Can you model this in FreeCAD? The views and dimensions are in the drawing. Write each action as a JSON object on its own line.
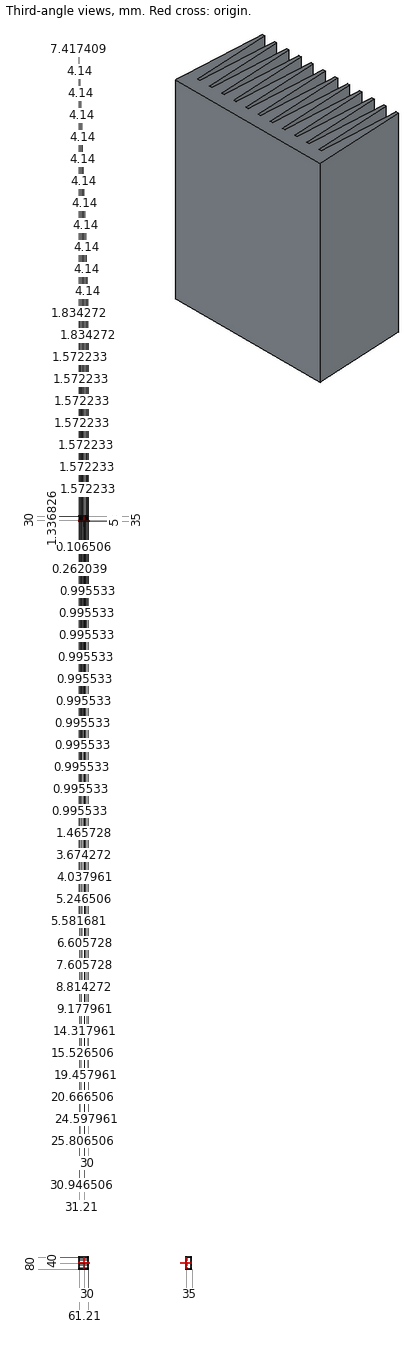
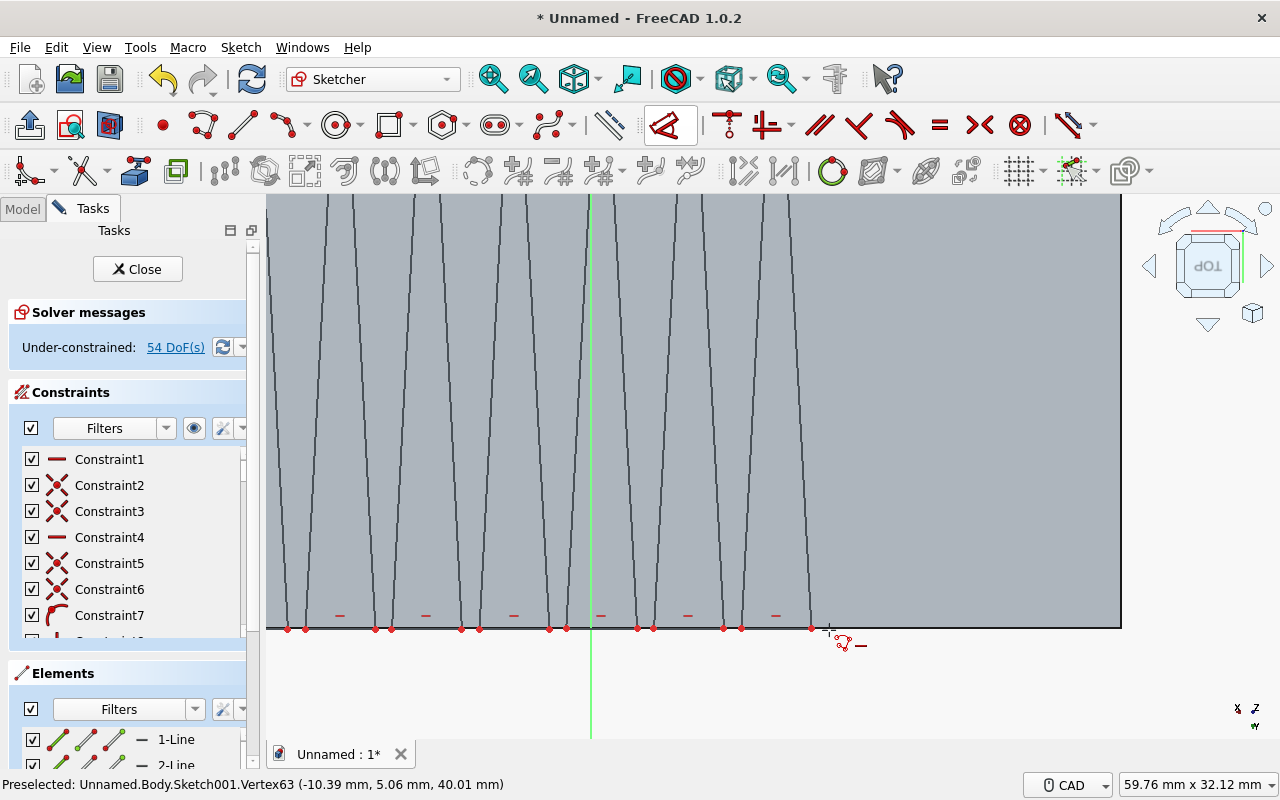
{"action": "left_click", "coordinate": [828, 628]}
{"action": "left_click", "coordinate": [898, 628]}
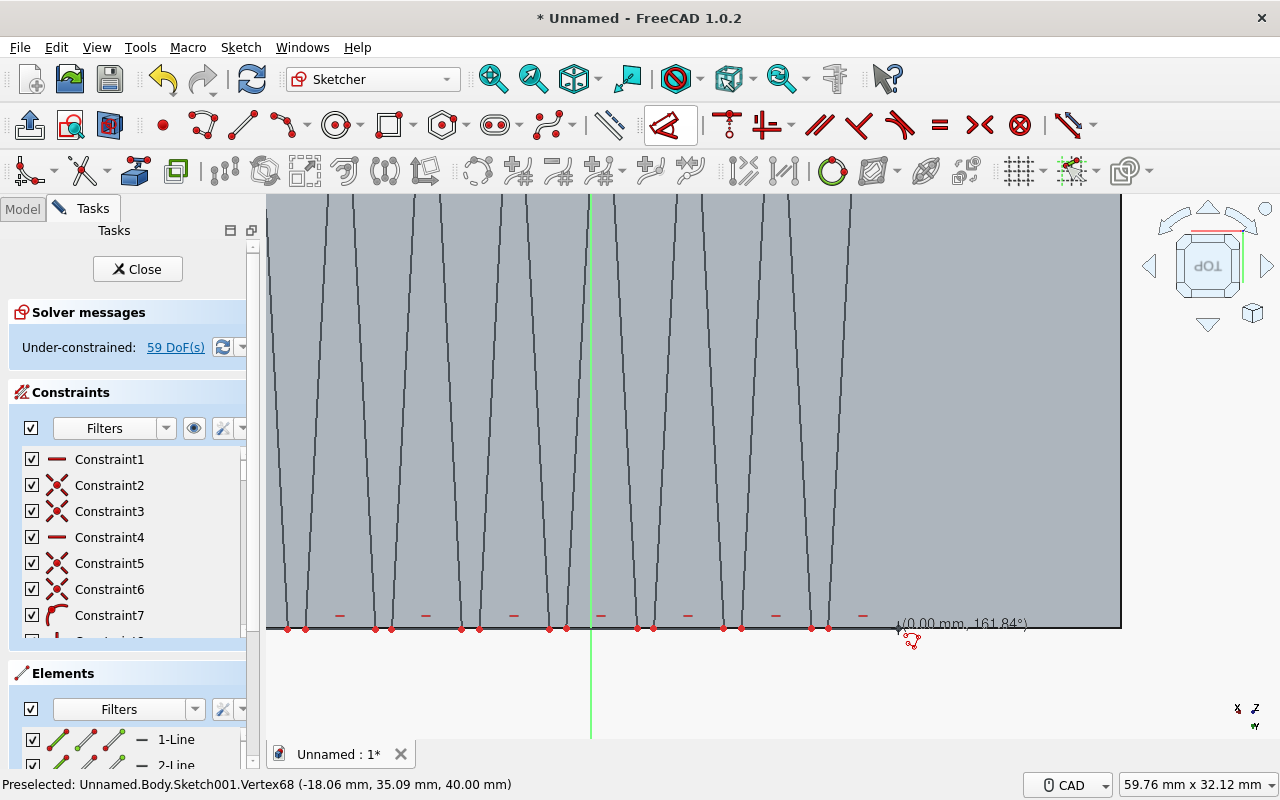
{"action": "scroll", "coordinate": [830, 631], "scroll_direction": "down", "scroll_amount": 3}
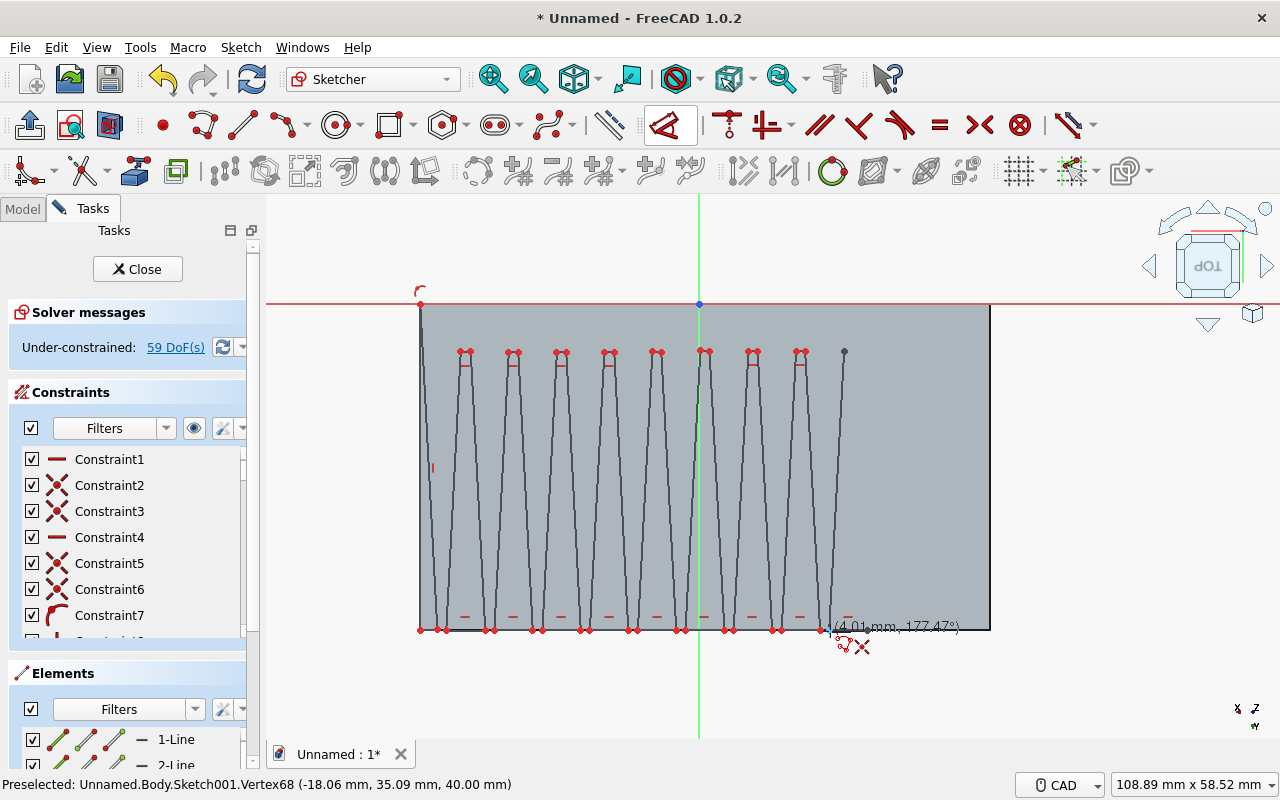
{"action": "scroll", "coordinate": [853, 351], "scroll_direction": "up", "scroll_amount": 3}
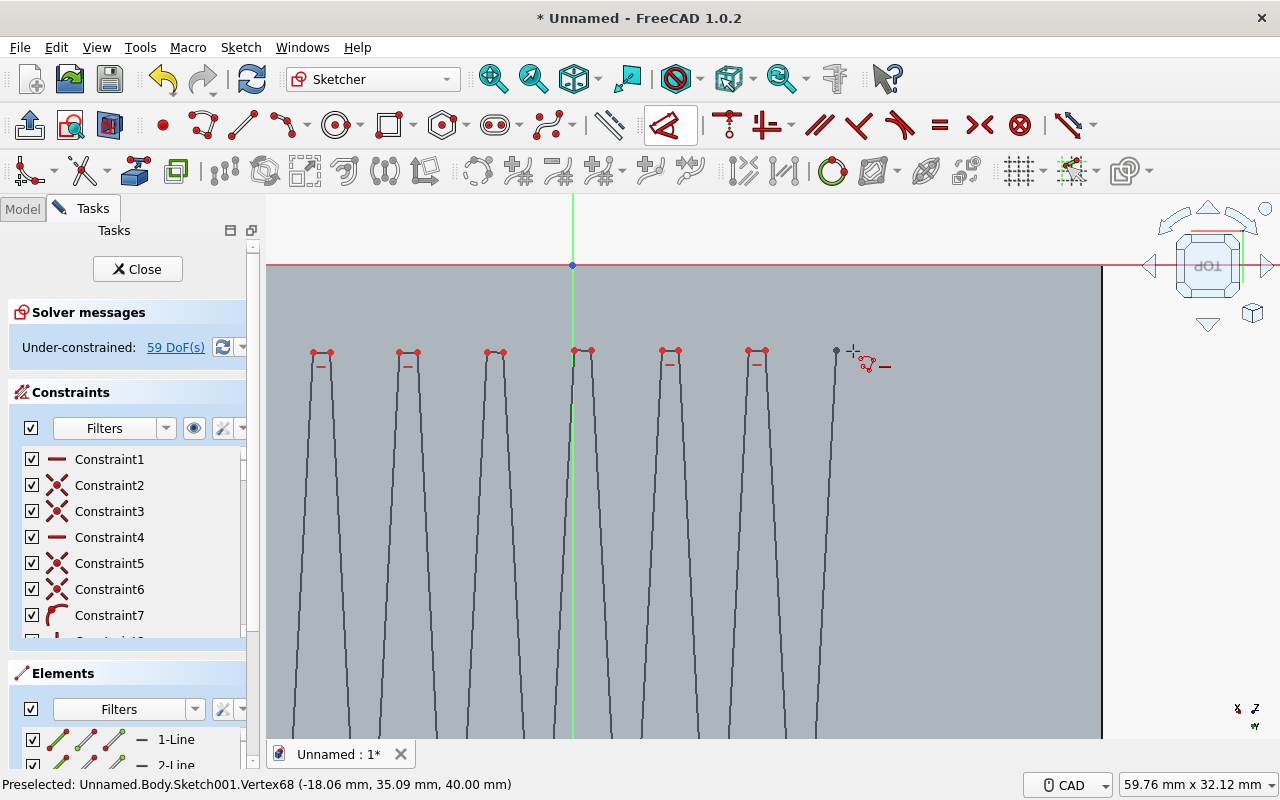
{"action": "left_click", "coordinate": [853, 350]}
{"action": "left_click", "coordinate": [836, 351]}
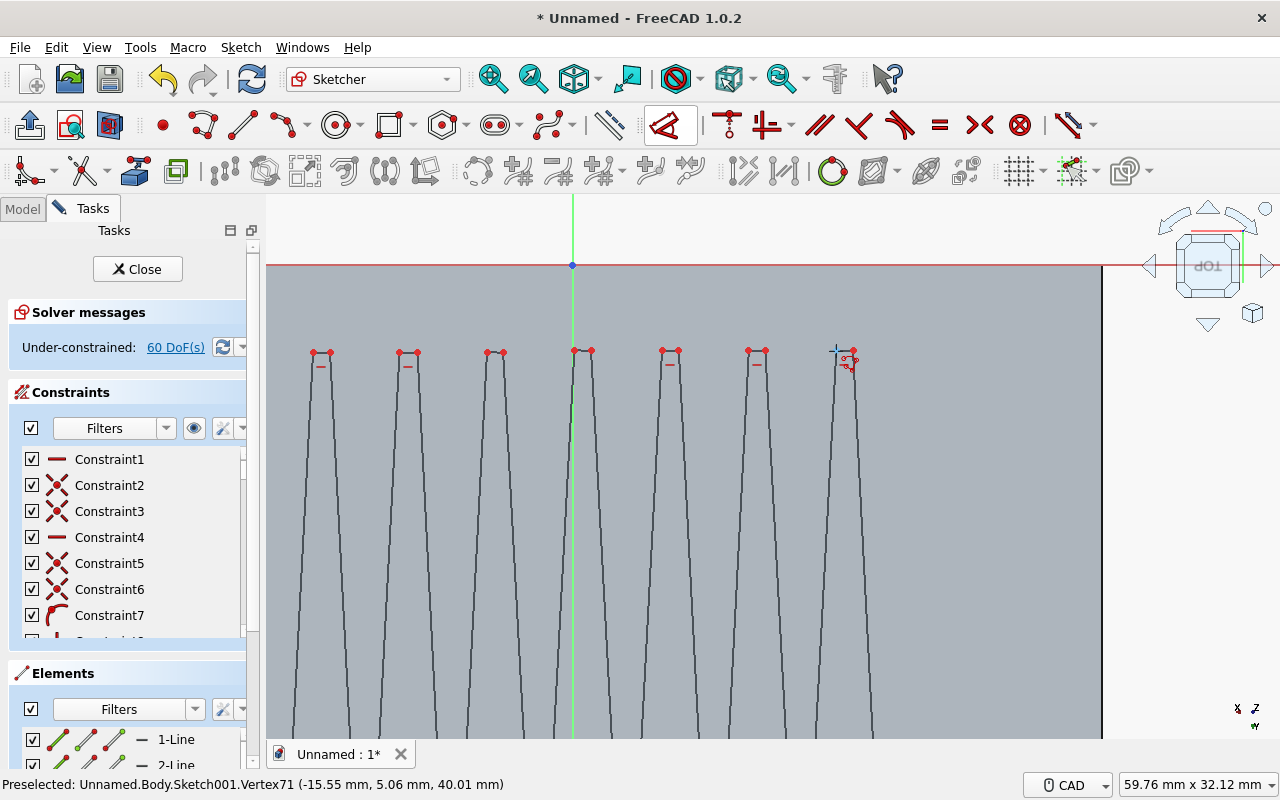
{"action": "left_click", "coordinate": [923, 350]}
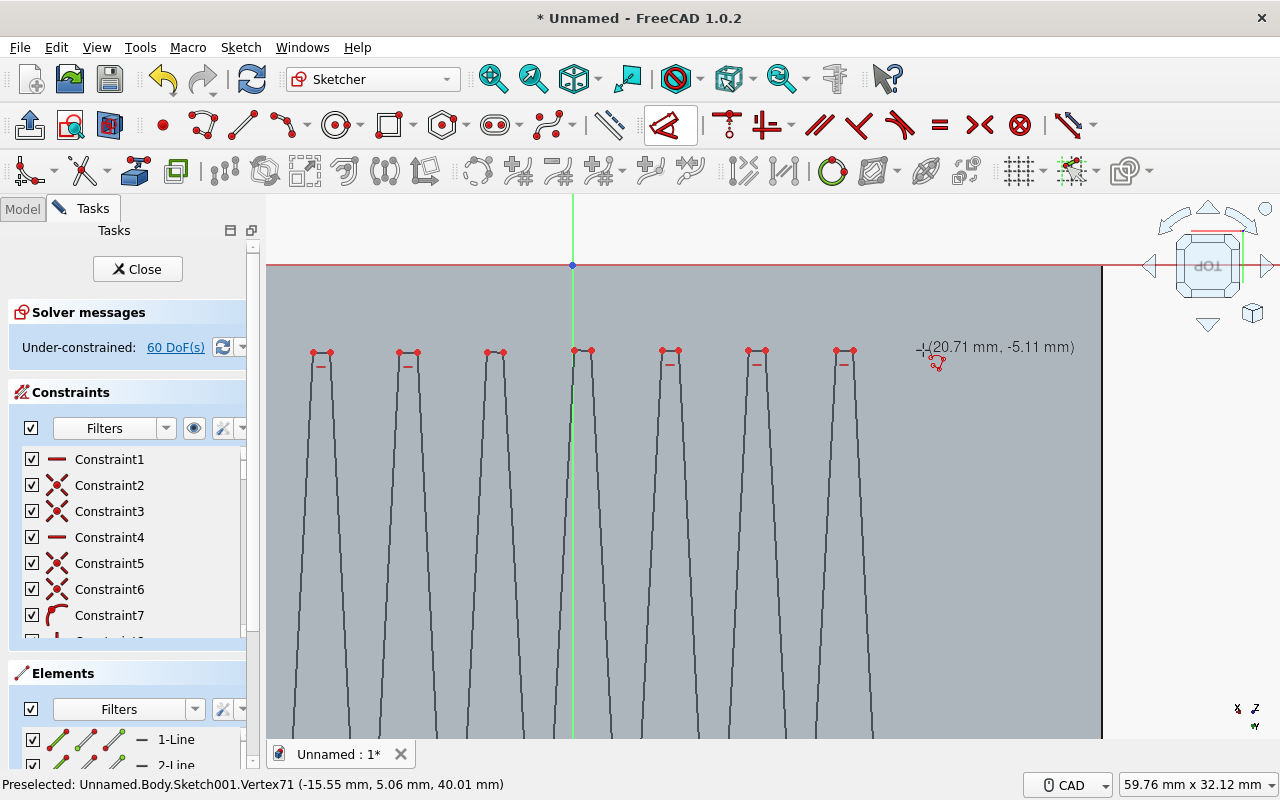
{"action": "scroll", "coordinate": [853, 350], "scroll_direction": "down", "scroll_amount": 3}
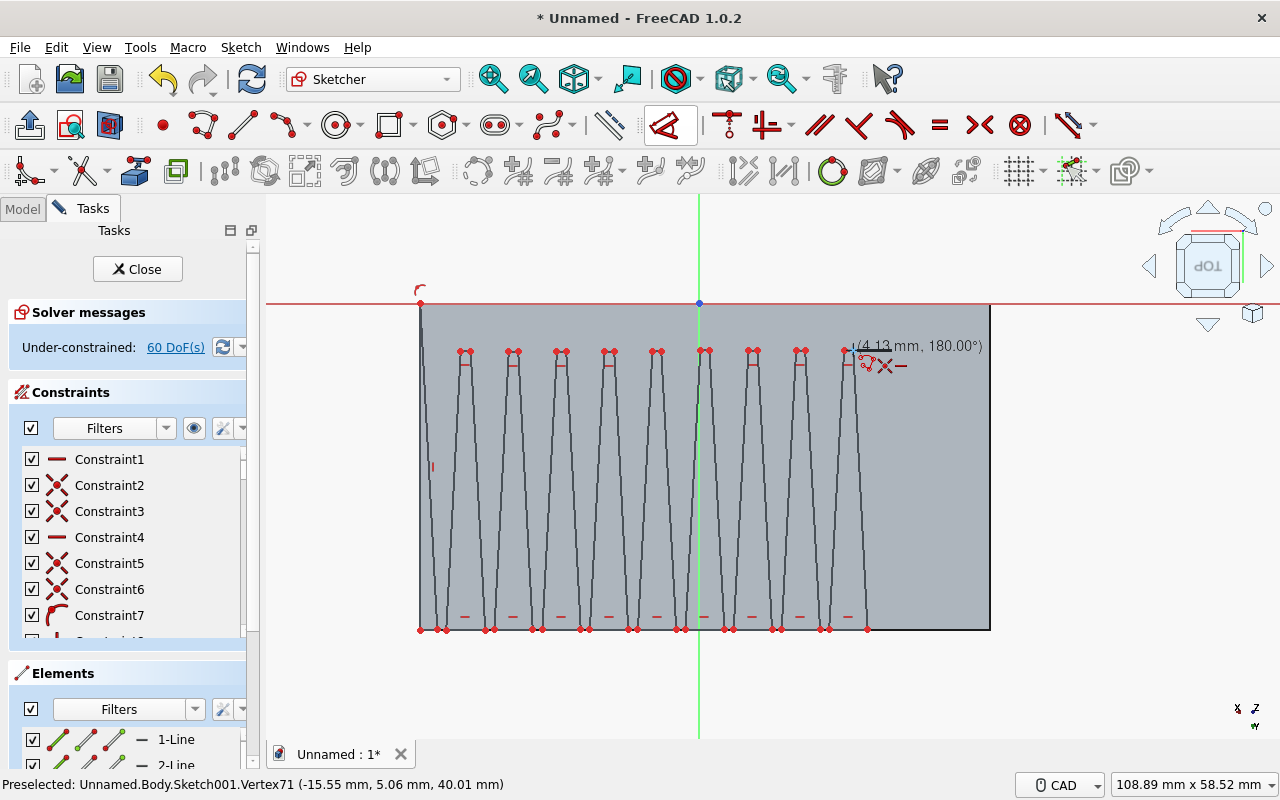
{"action": "scroll", "coordinate": [877, 630], "scroll_direction": "up", "scroll_amount": 3}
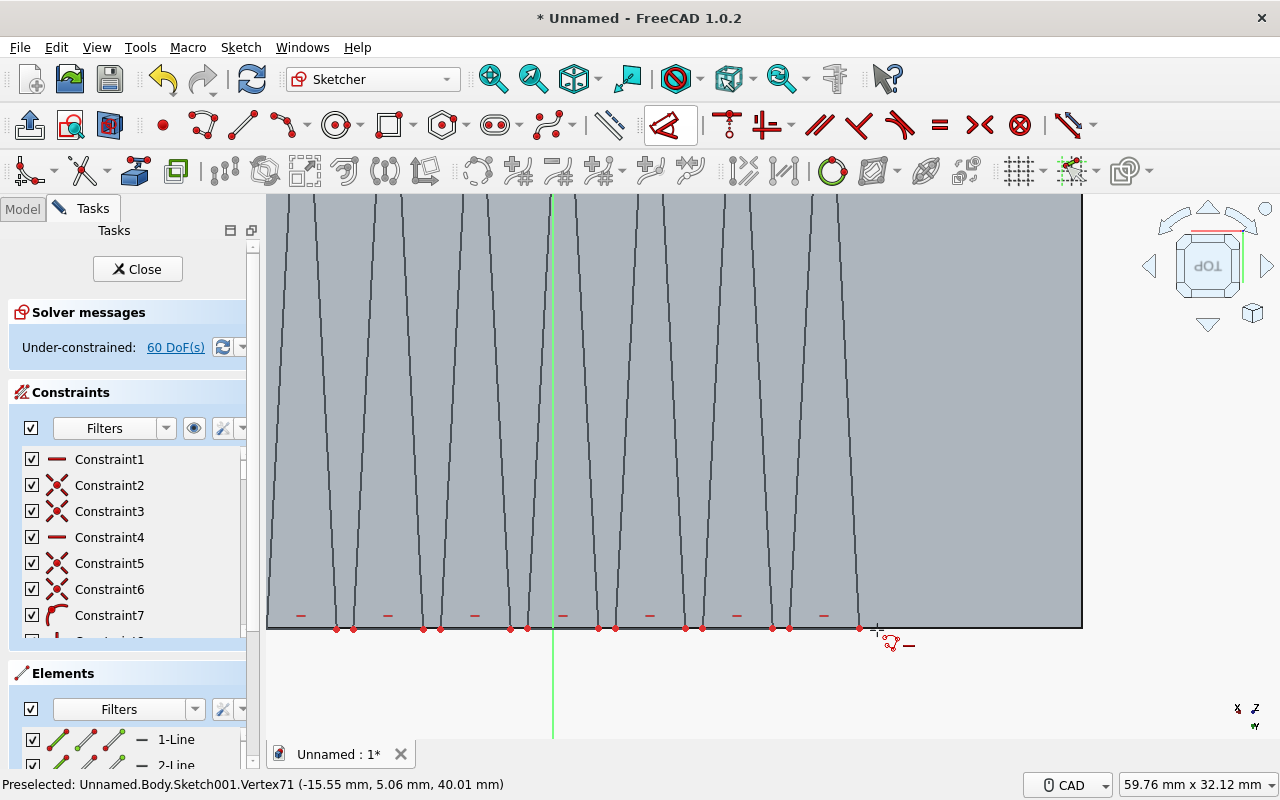
{"action": "left_click", "coordinate": [877, 628]}
{"action": "left_click", "coordinate": [947, 628]}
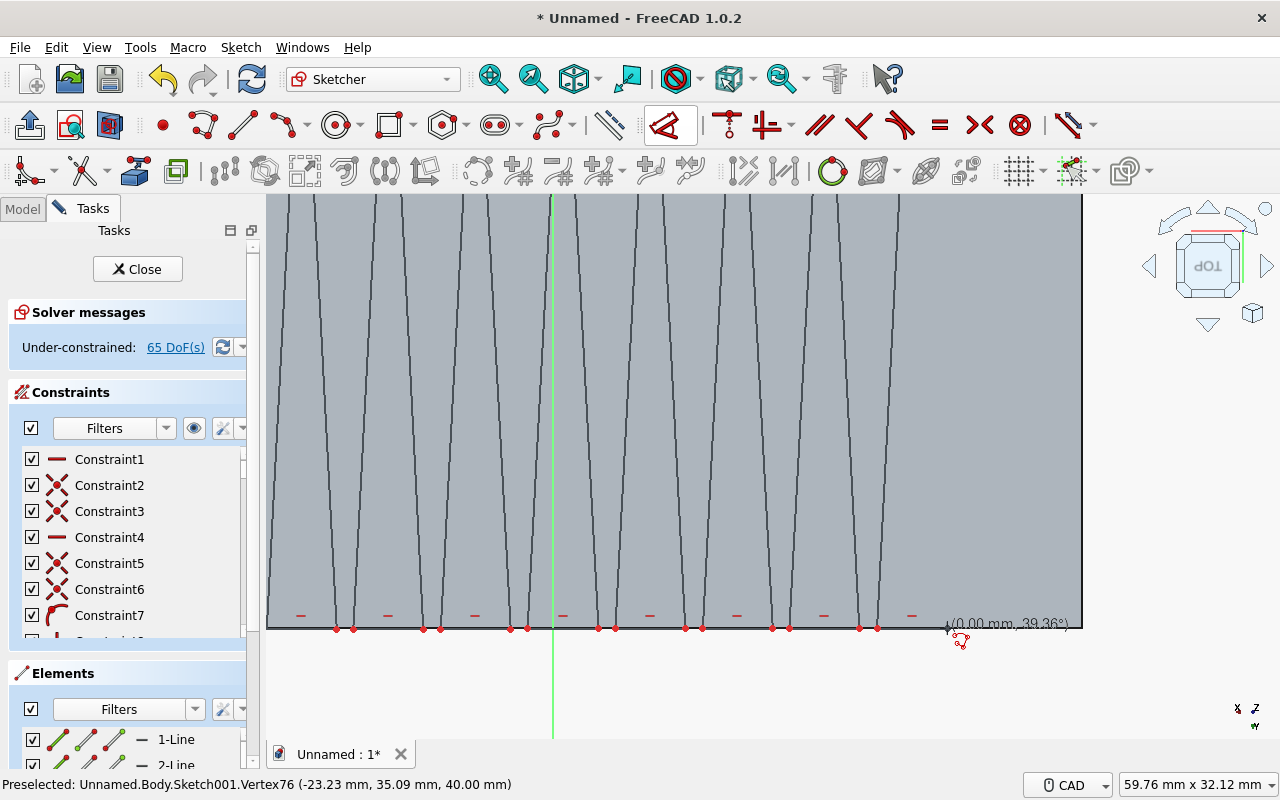
{"action": "scroll", "coordinate": [877, 631], "scroll_direction": "down", "scroll_amount": 3}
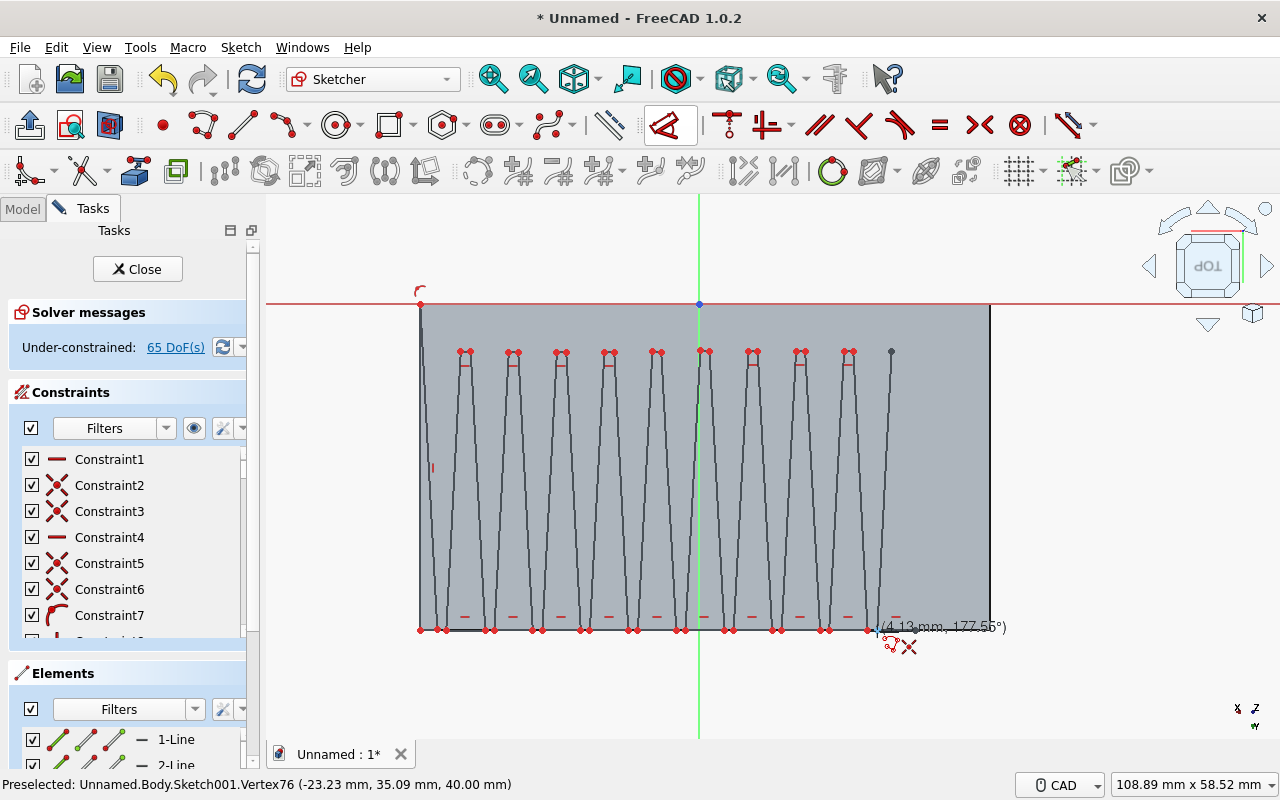
{"action": "scroll", "coordinate": [901, 351], "scroll_direction": "up", "scroll_amount": 3}